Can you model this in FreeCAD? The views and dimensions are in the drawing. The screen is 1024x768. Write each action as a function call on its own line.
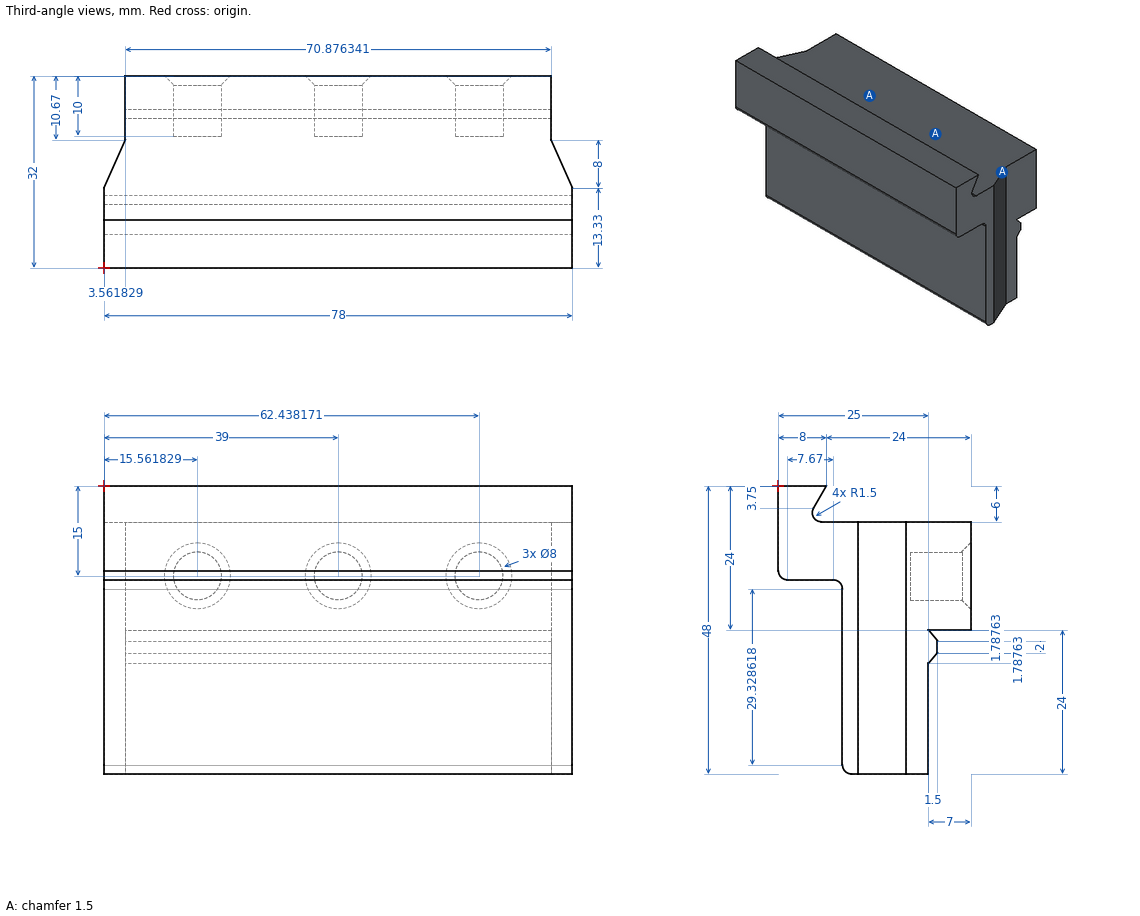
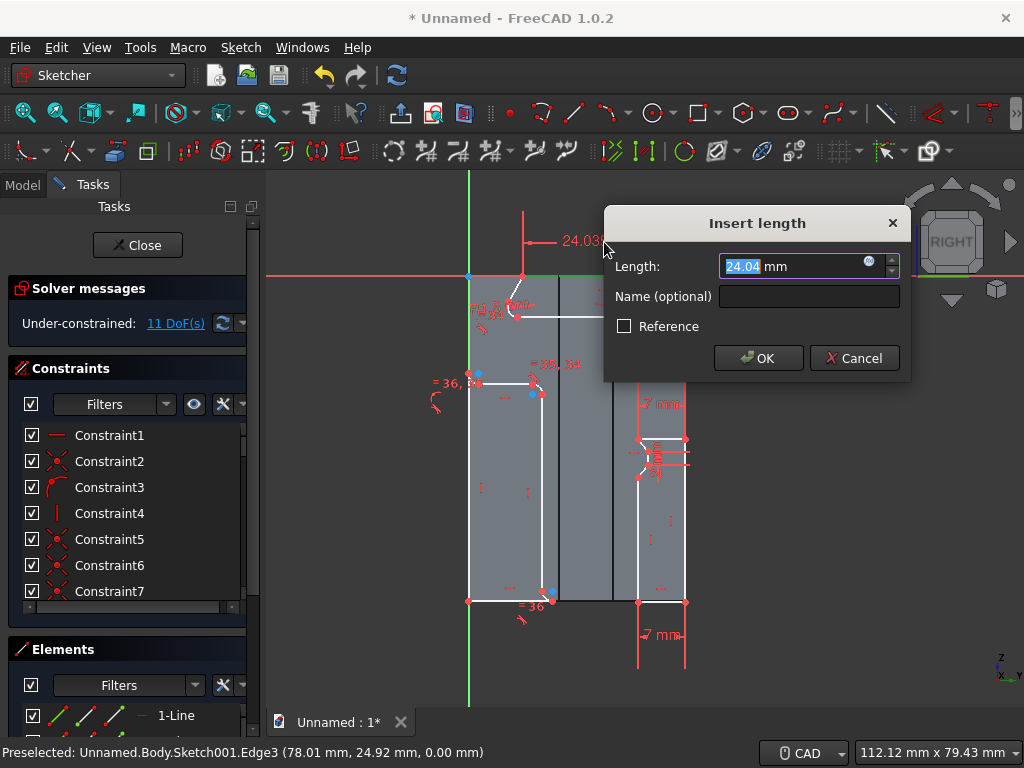
text(24)
key(Return)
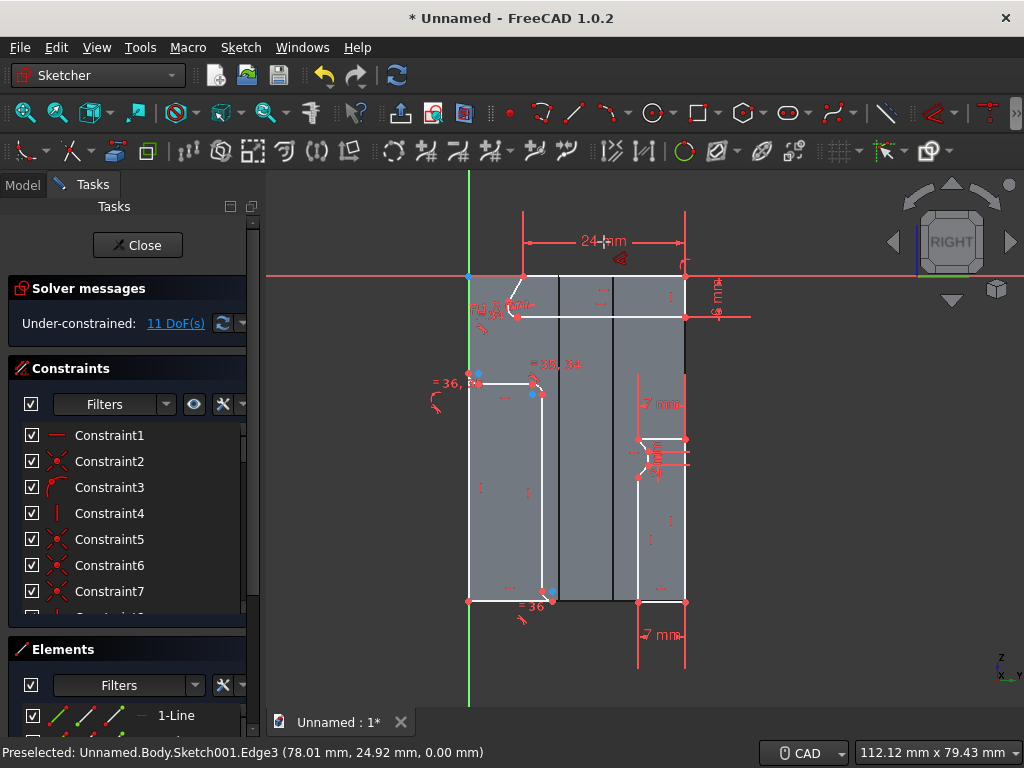
click(685, 553)
click(719, 521)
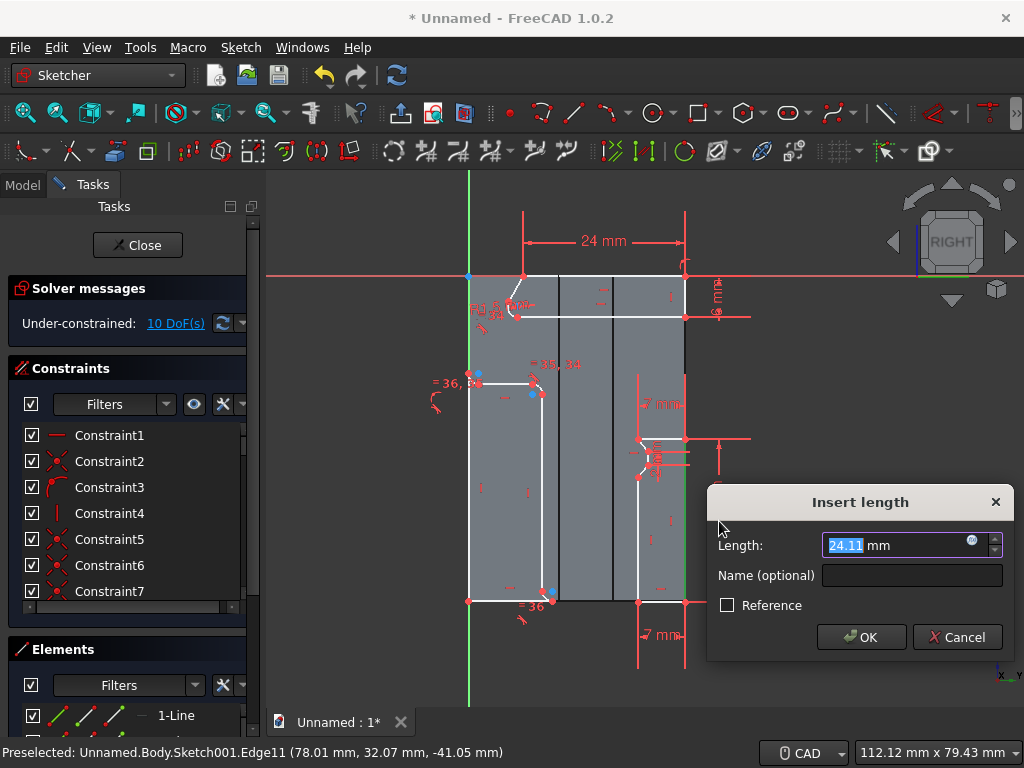
text(24)
key(Return)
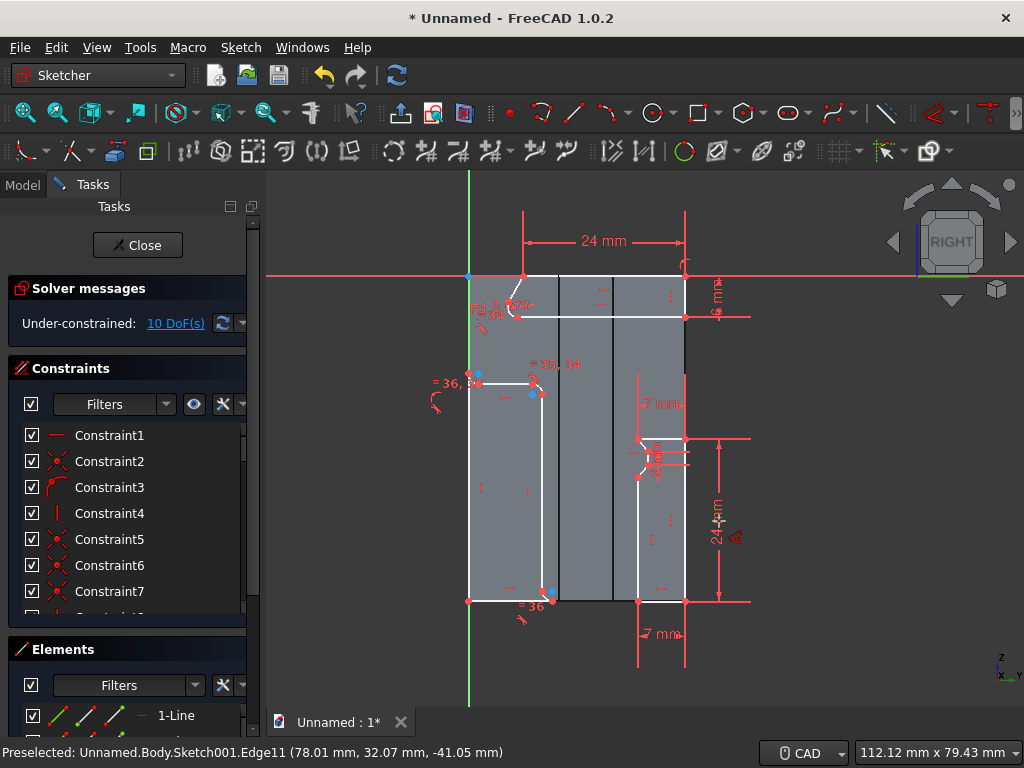
click(523, 276)
click(496, 242)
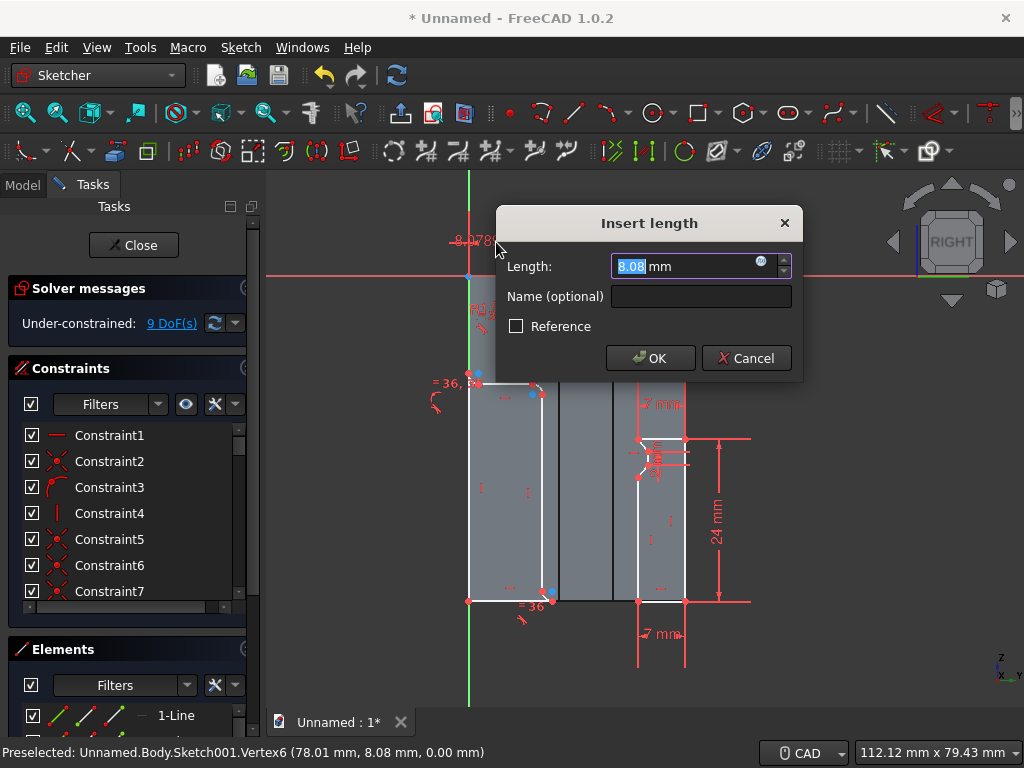
text(8)
key(Return)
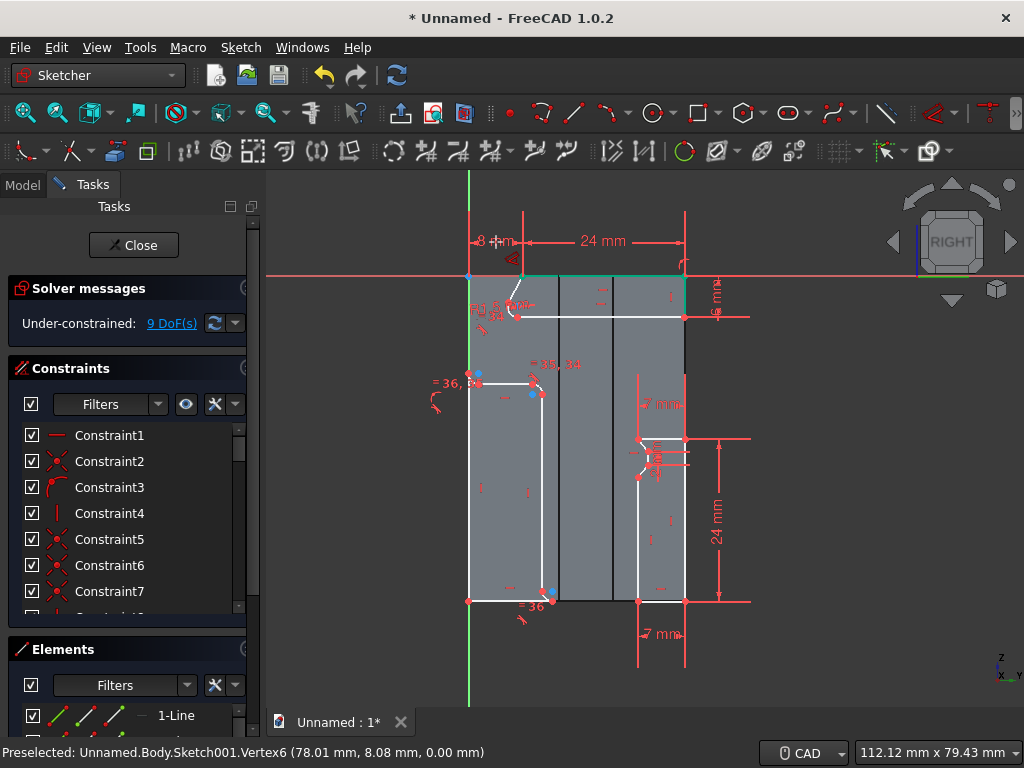
click(638, 439)
click(514, 473)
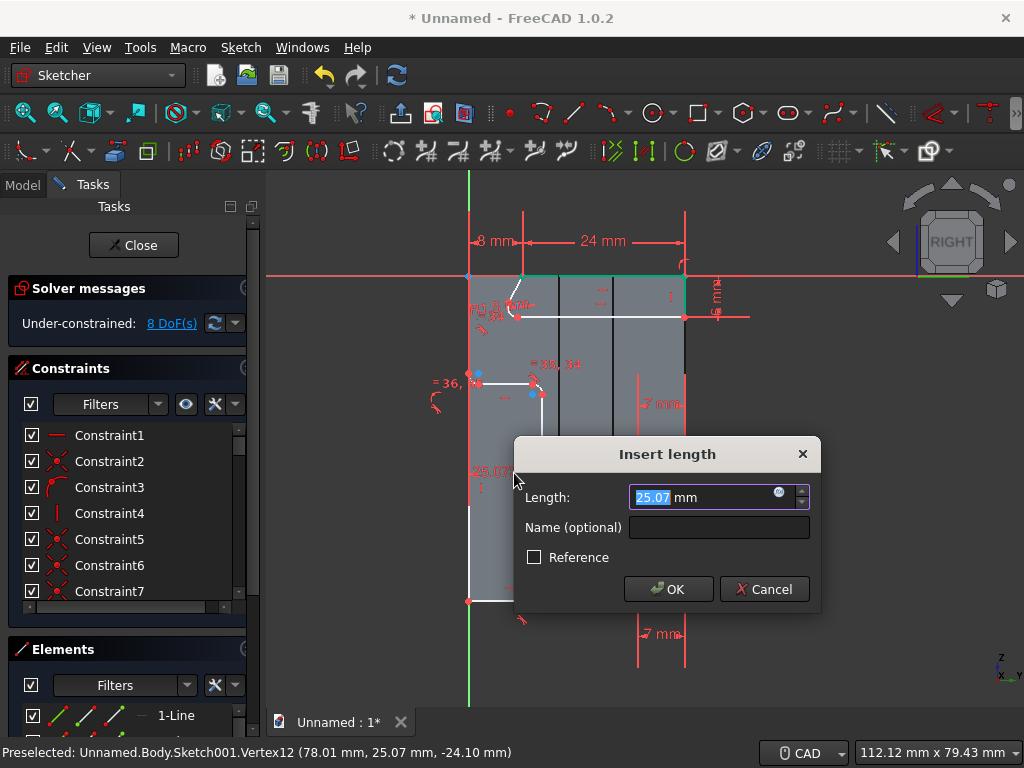
text(25)
key(Return)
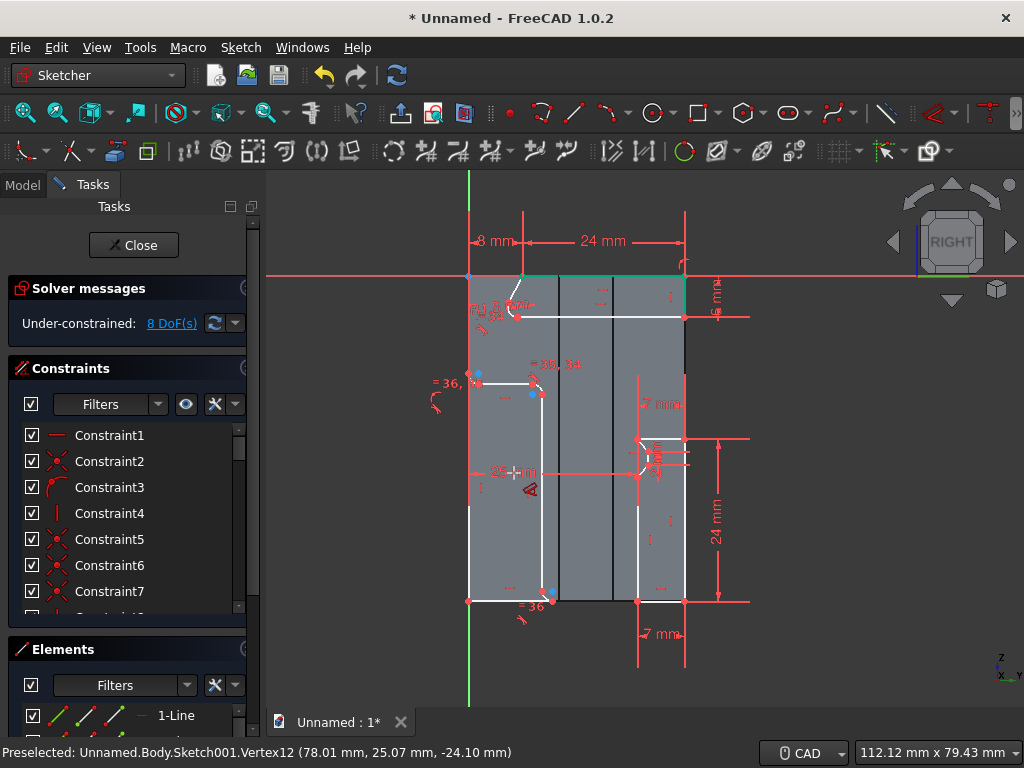
click(638, 439)
click(435, 358)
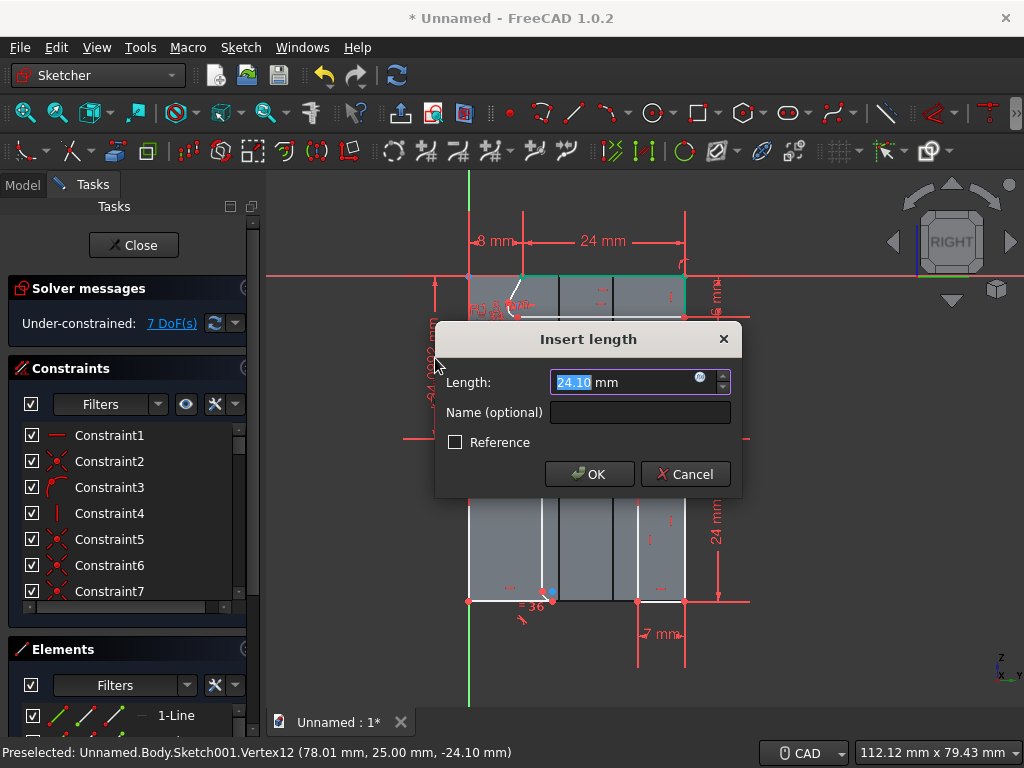
text(24)
key(Return)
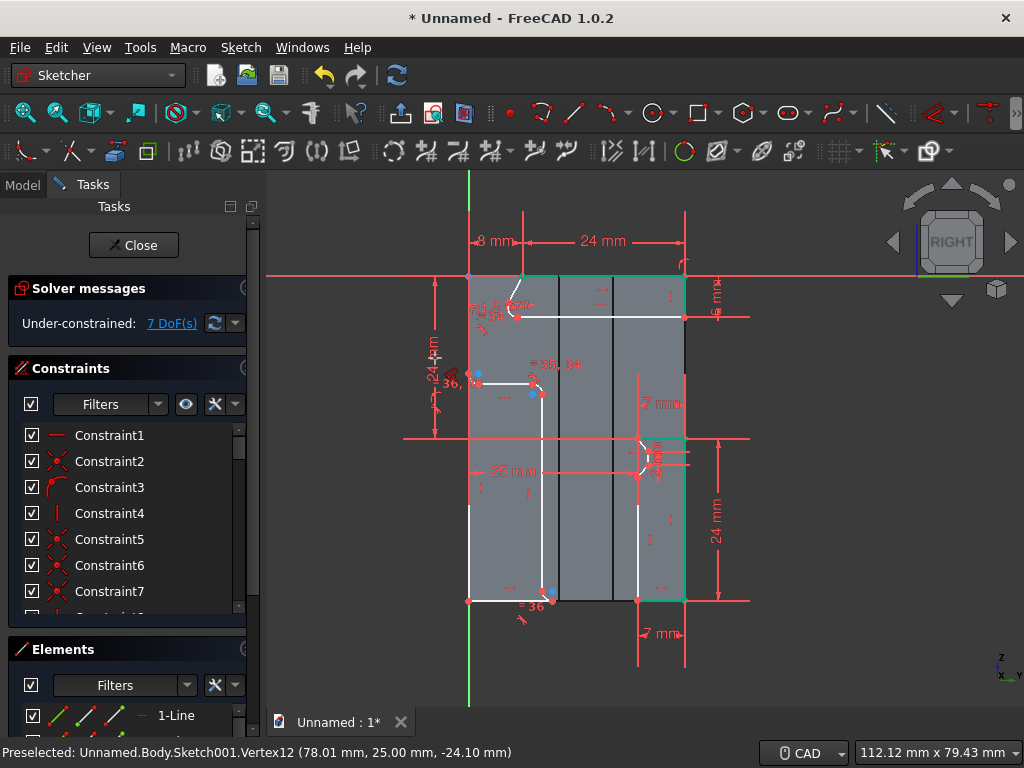
click(469, 601)
click(435, 439)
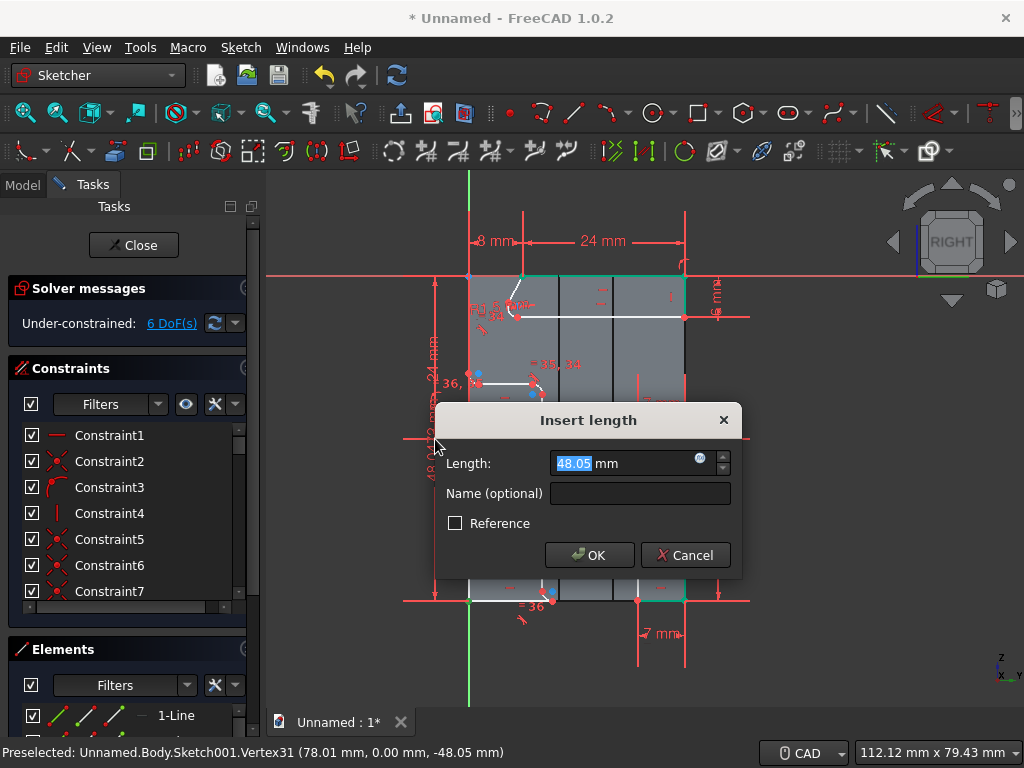
text(48)
key(Return)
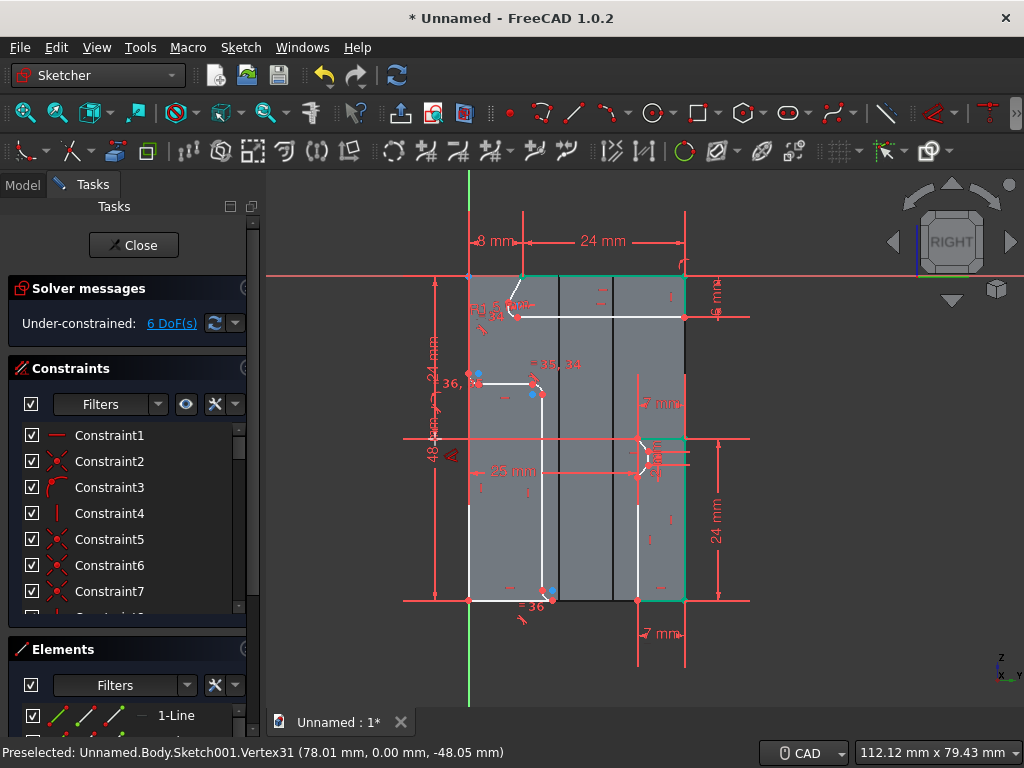
click(516, 384)
click(505, 350)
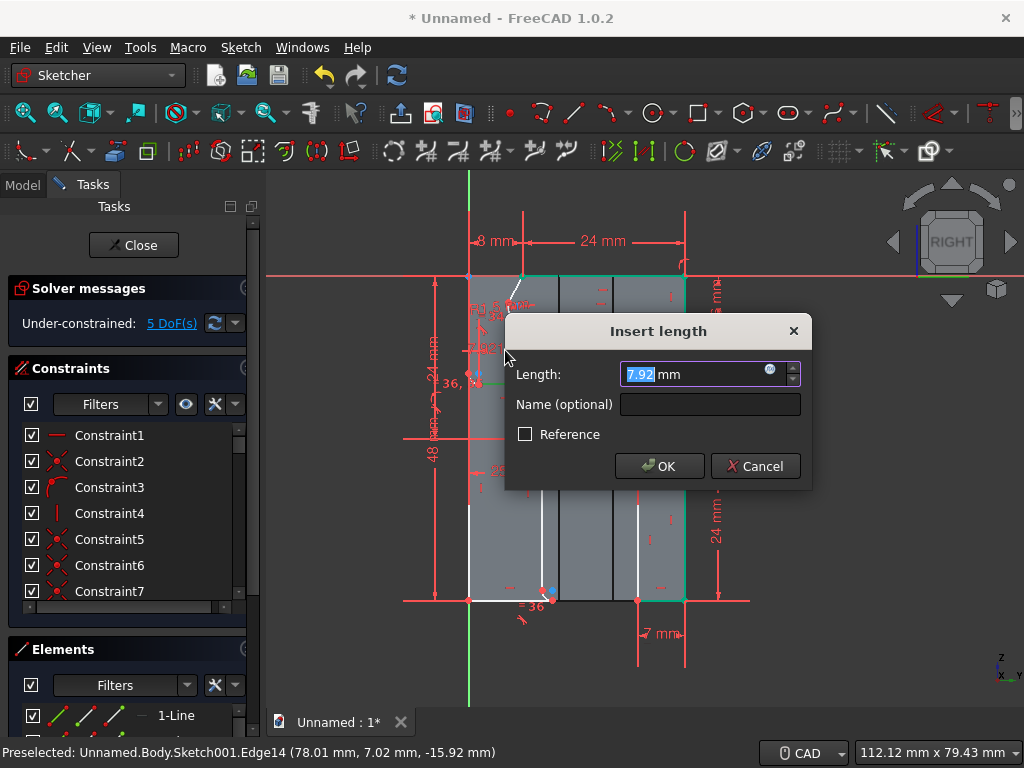
text(7.67)
key(Return)